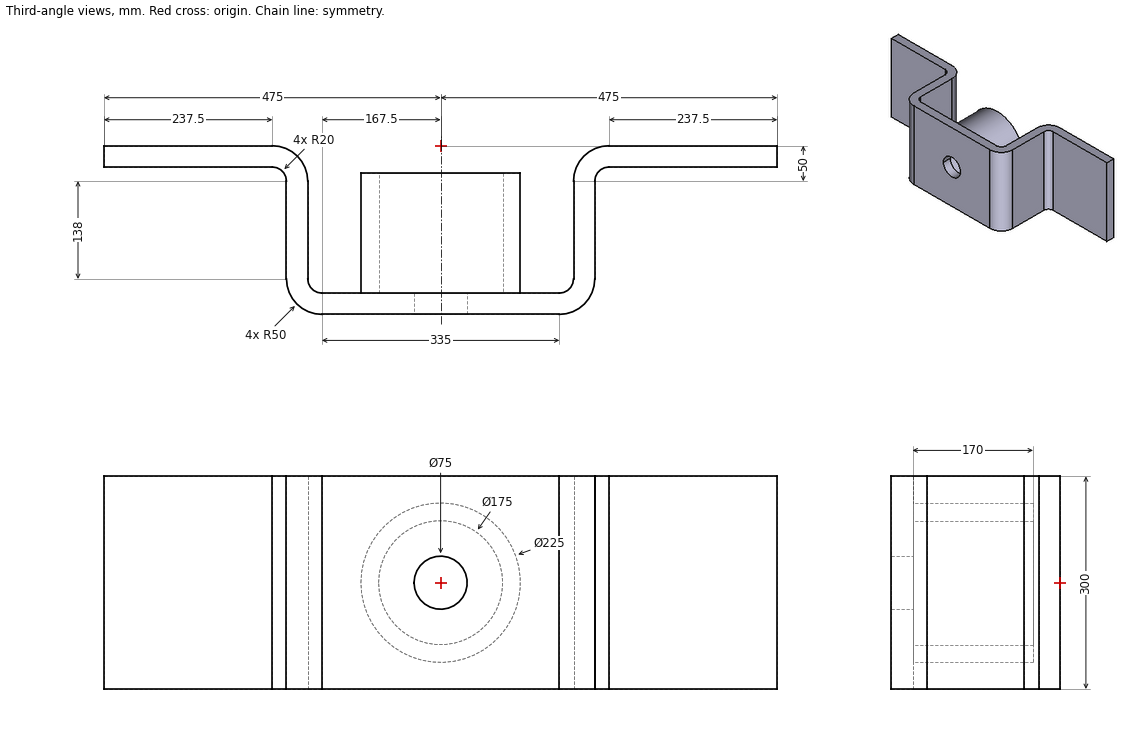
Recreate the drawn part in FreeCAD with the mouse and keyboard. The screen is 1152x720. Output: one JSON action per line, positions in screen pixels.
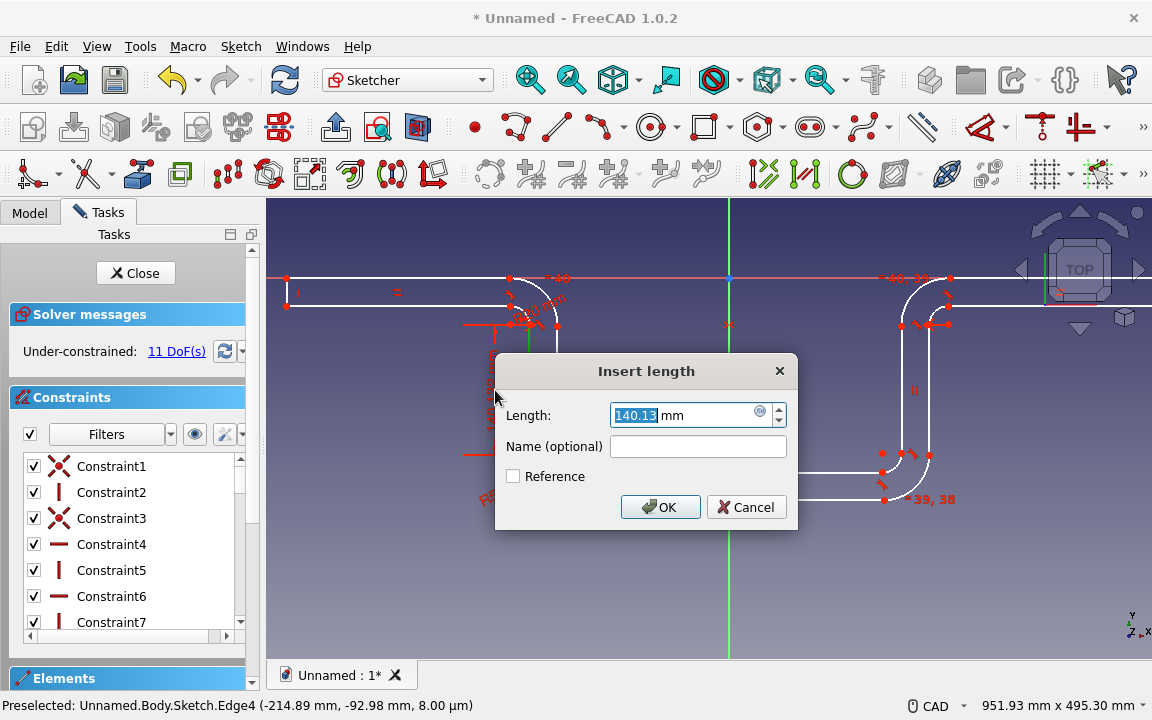
{"action": "type", "text": "138"}
{"action": "key", "text": "Return"}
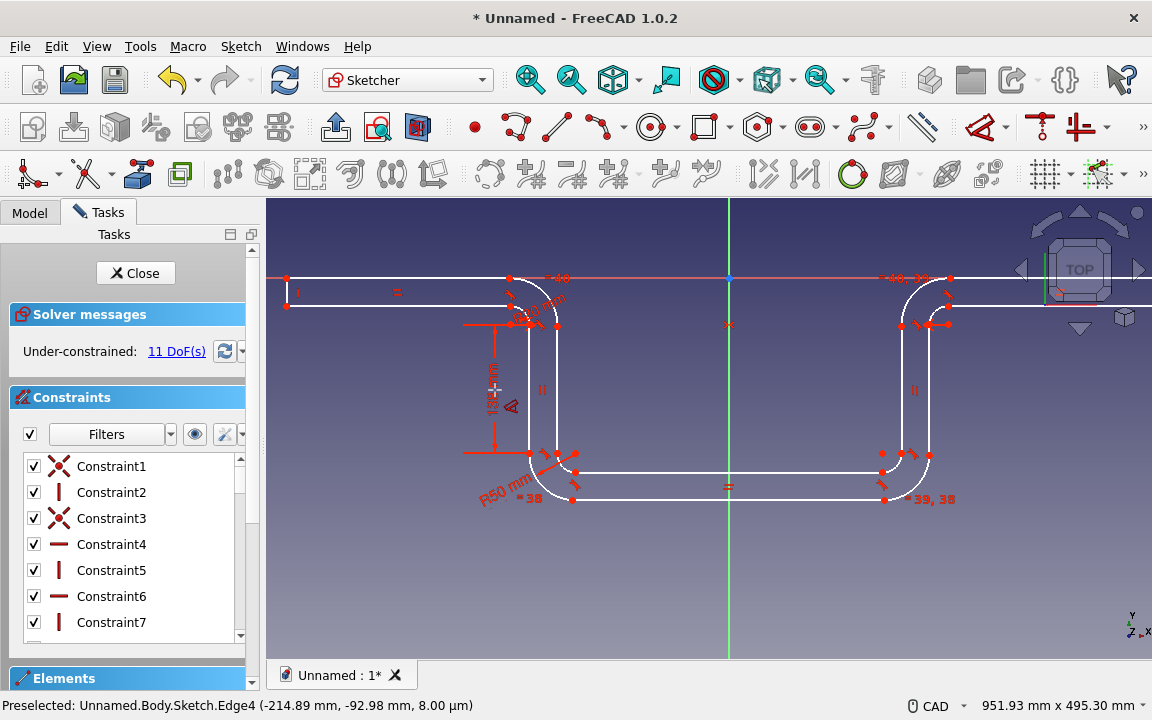
{"action": "left_click", "coordinate": [666, 500]}
{"action": "left_click", "coordinate": [657, 534]}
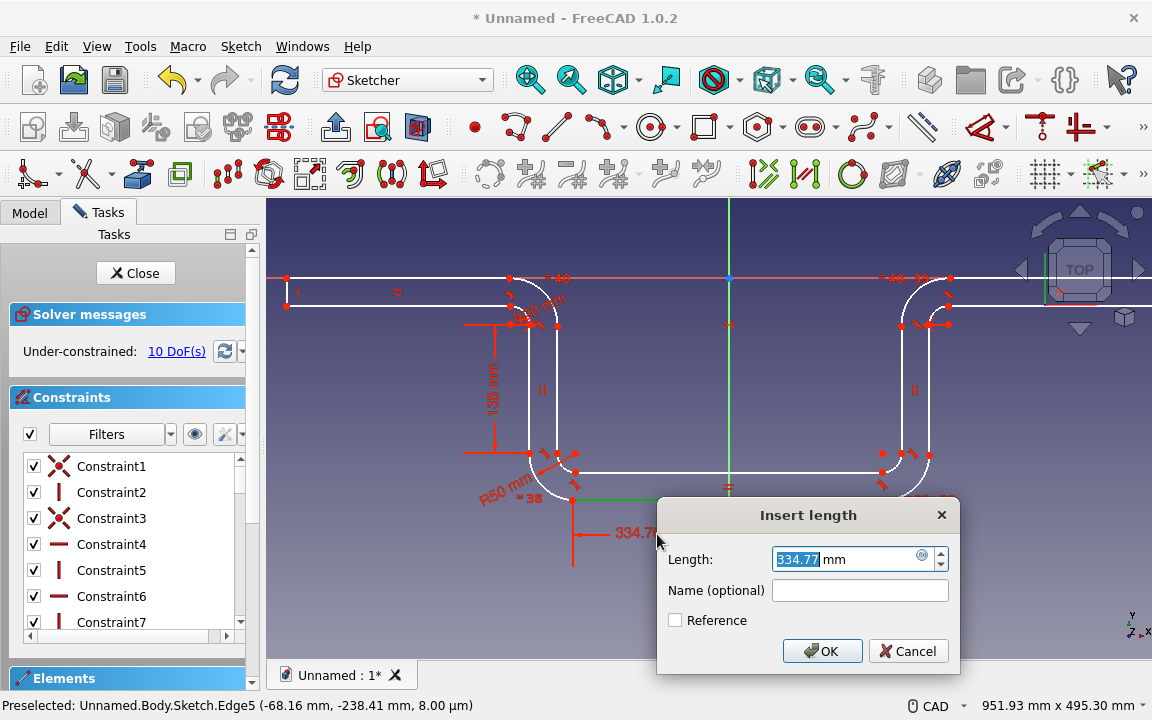
{"action": "type", "text": "335"}
{"action": "key", "text": "Return"}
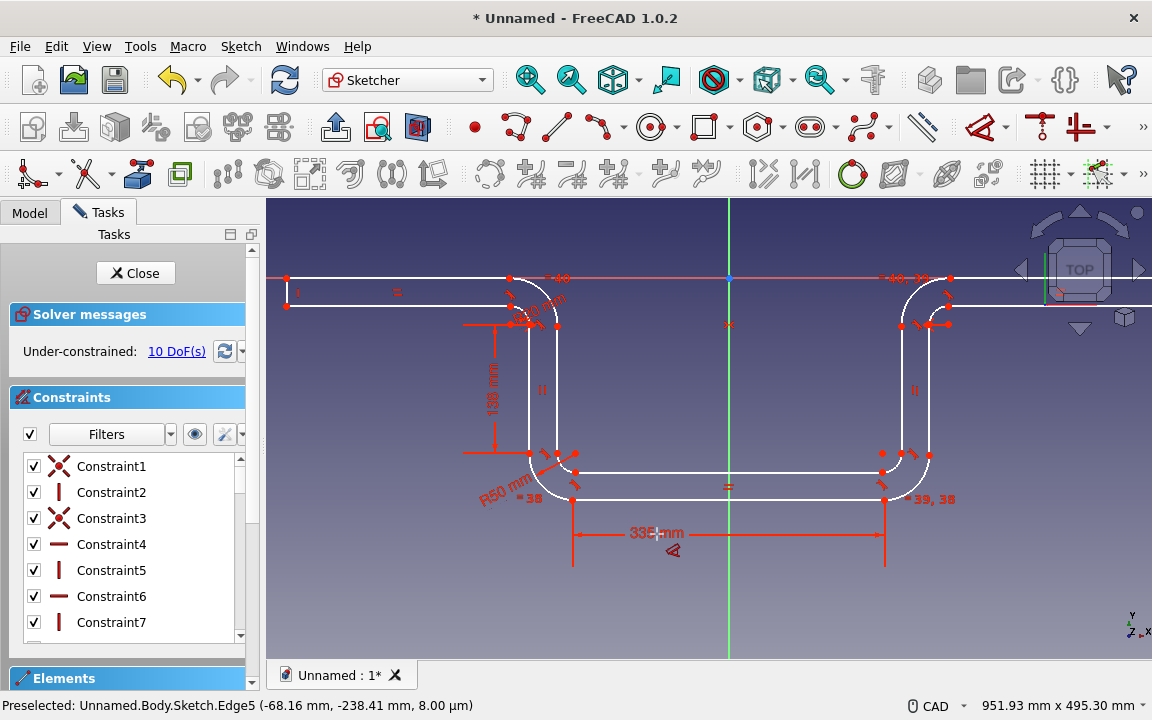
{"action": "left_click", "coordinate": [929, 416]}
{"action": "left_click", "coordinate": [963, 390]}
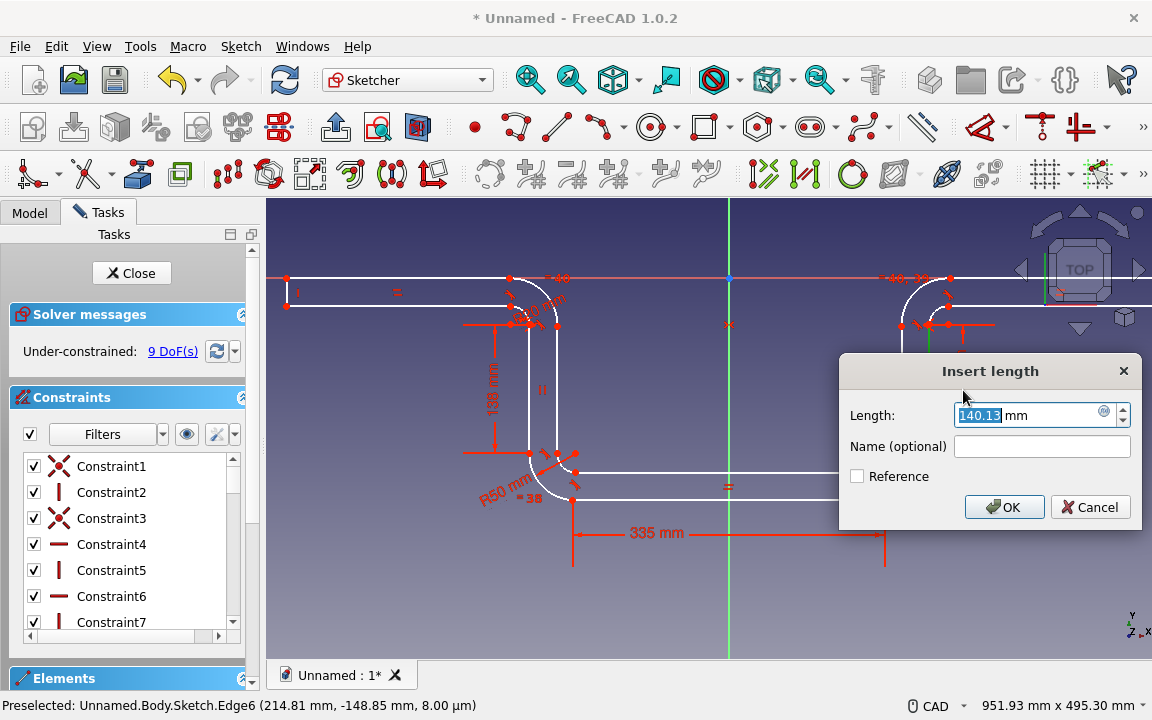
{"action": "type", "text": "138"}
{"action": "key", "text": "Return"}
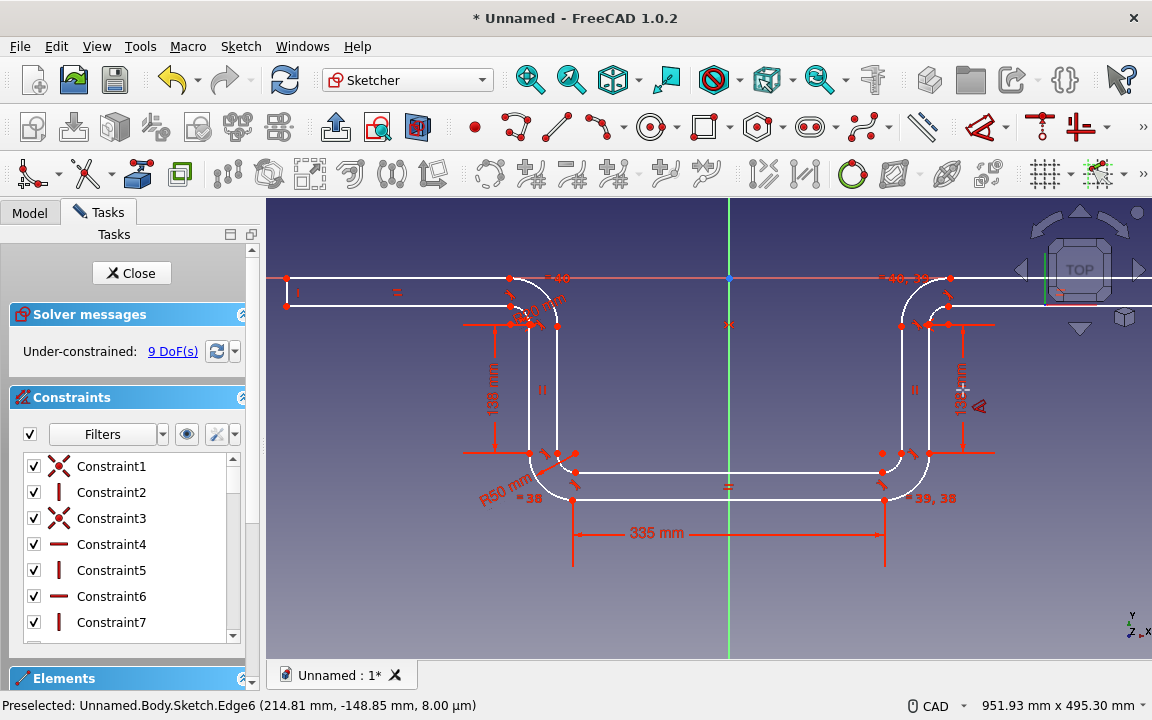
{"action": "left_click", "coordinate": [902, 364]}
{"action": "left_click", "coordinate": [868, 390]}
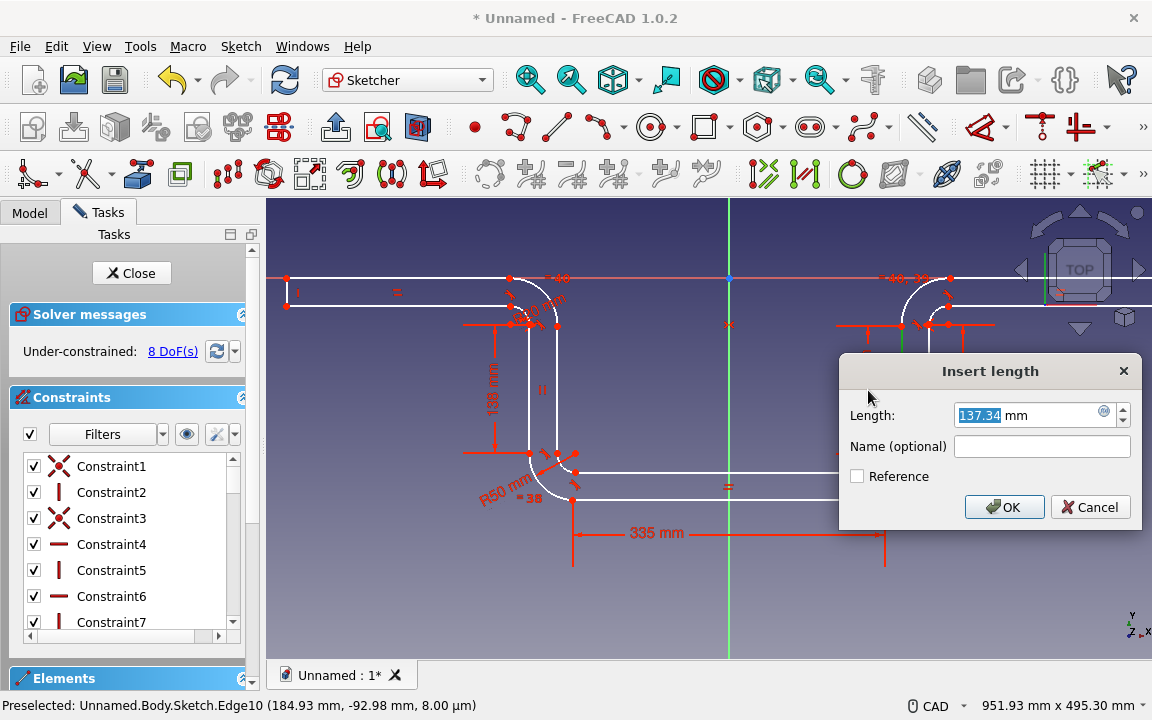
{"action": "type", "text": "138"}
{"action": "key", "text": "Return"}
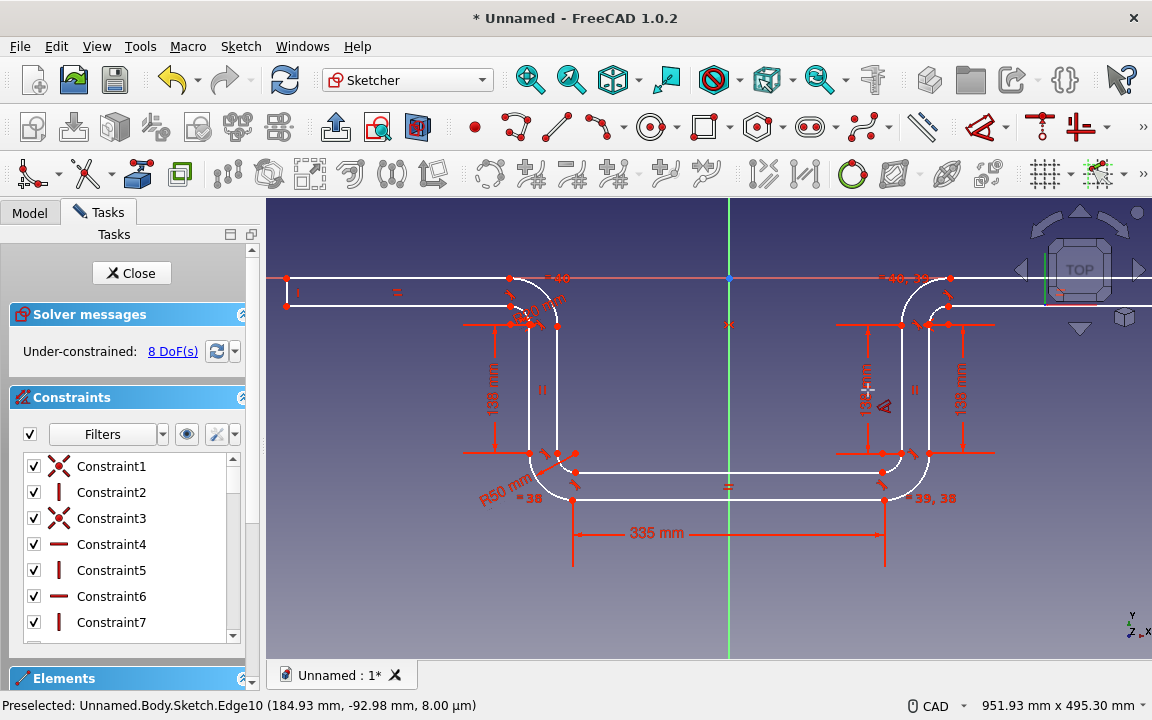
{"action": "left_click", "coordinate": [791, 473]}
{"action": "left_click", "coordinate": [659, 439]}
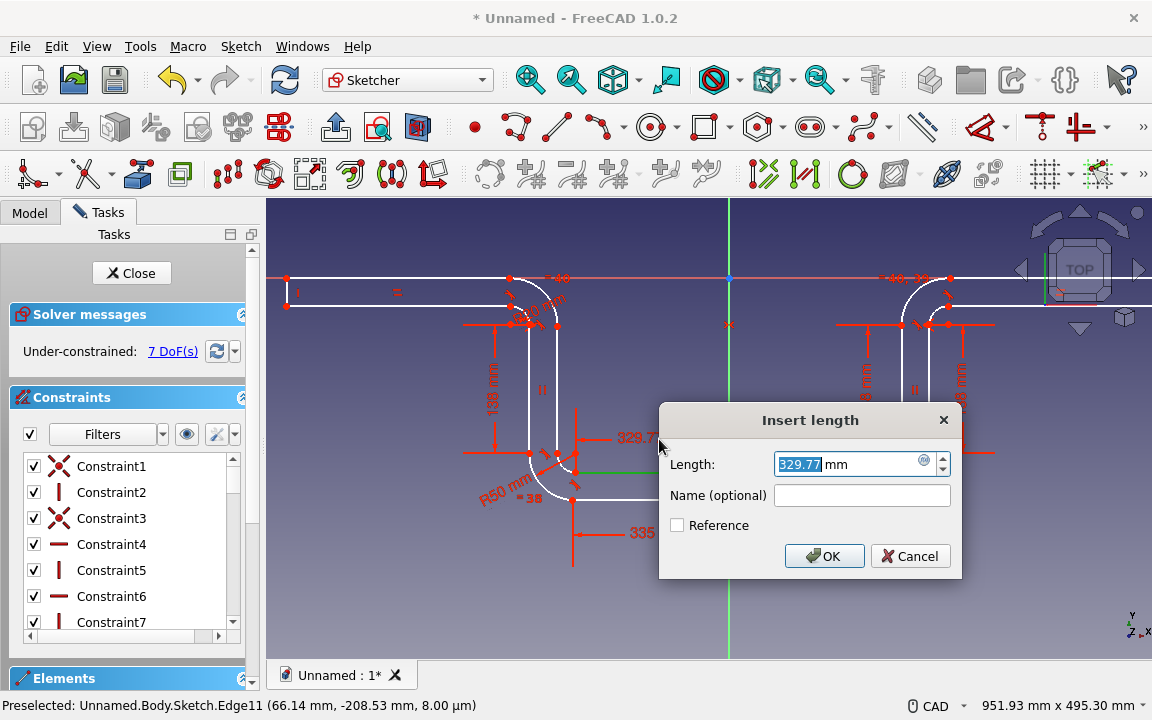
{"action": "type", "text": "335"}
{"action": "key", "text": "Return"}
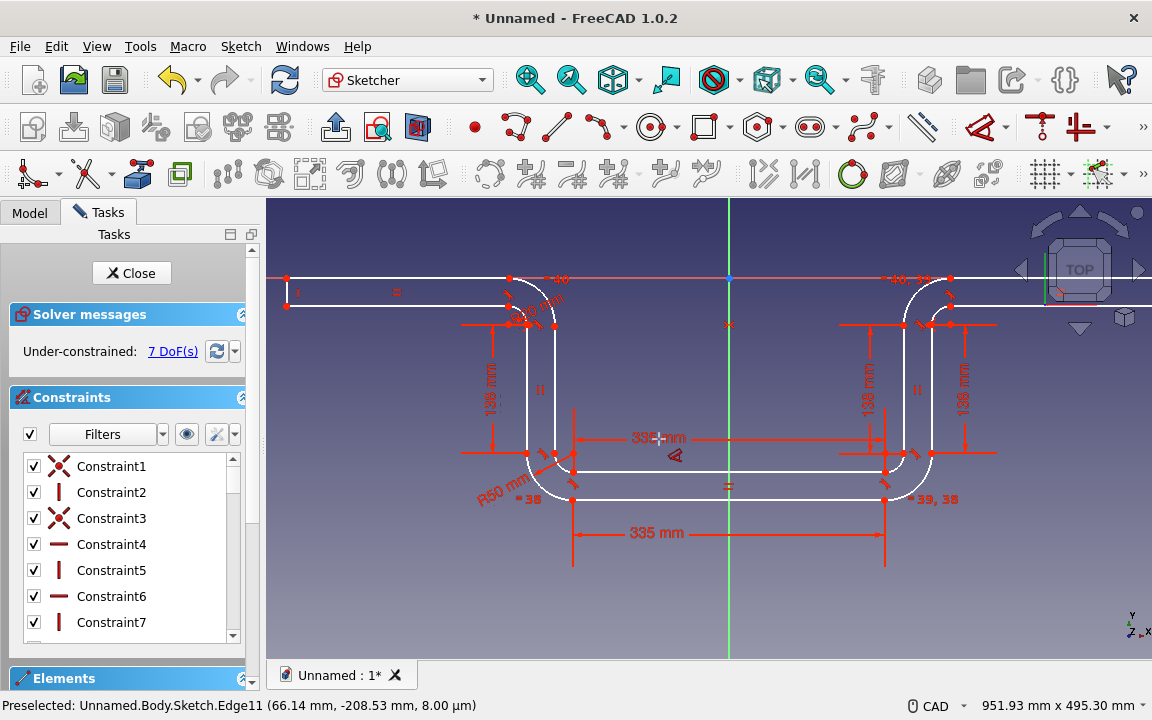
{"action": "left_click", "coordinate": [555, 415]}
{"action": "left_click", "coordinate": [589, 390]}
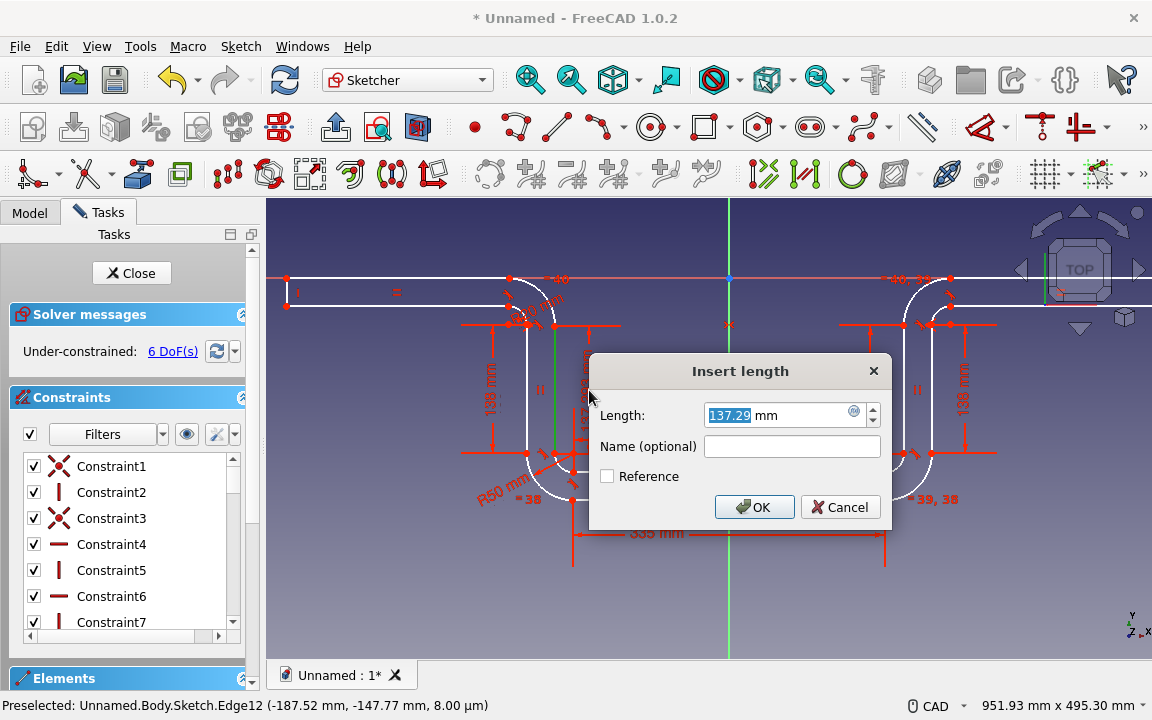
{"action": "type", "text": "138"}
{"action": "key", "text": "Return"}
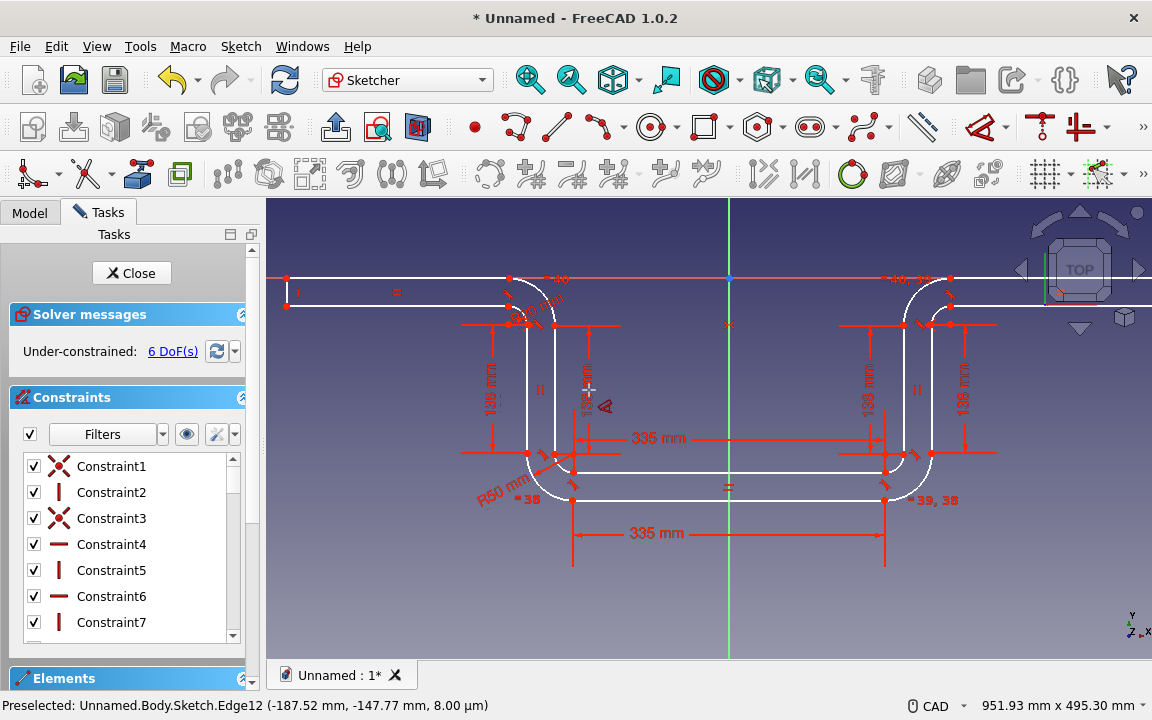
{"action": "left_click", "coordinate": [904, 326]}
{"action": "left_click", "coordinate": [695, 302]}